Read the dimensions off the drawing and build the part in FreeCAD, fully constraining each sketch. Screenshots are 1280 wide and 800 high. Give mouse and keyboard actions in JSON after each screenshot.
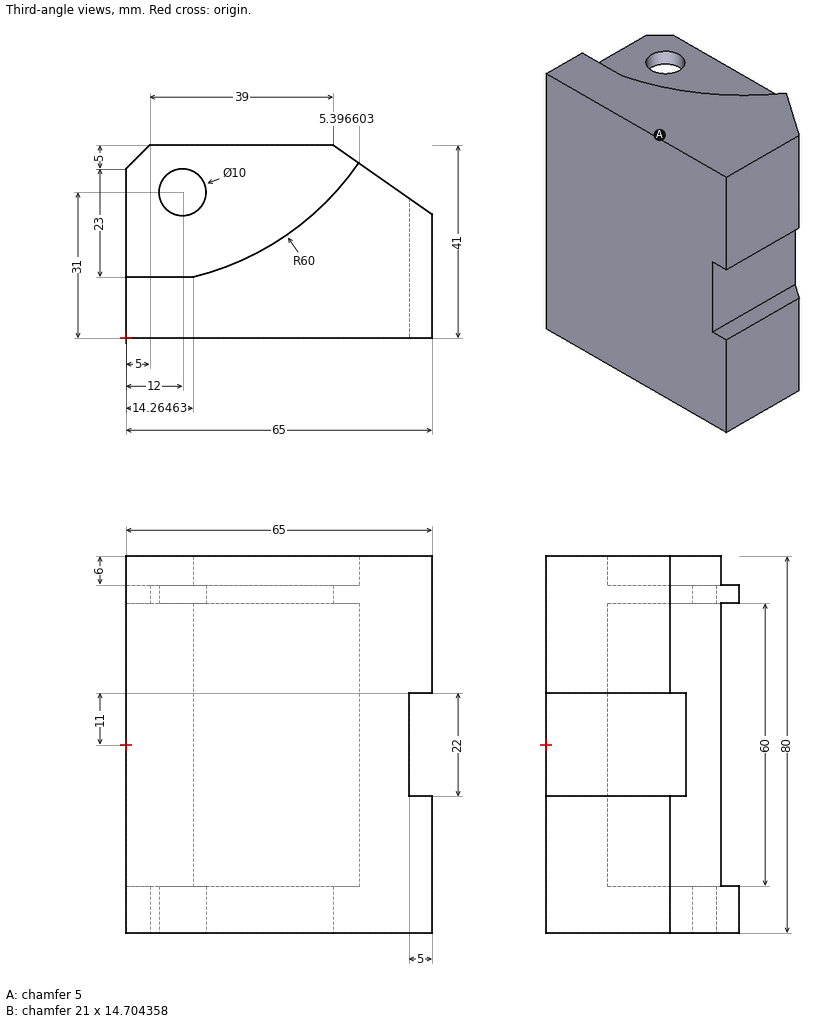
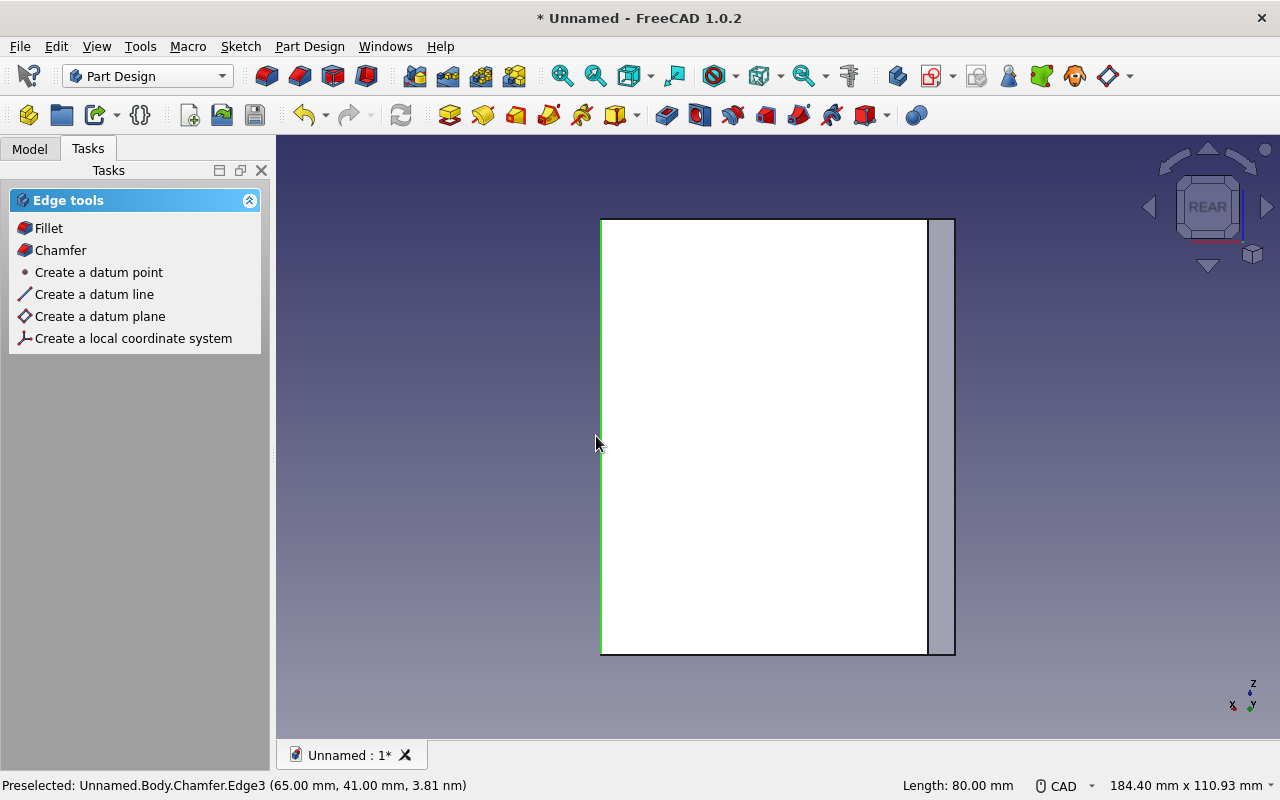
{"action": "left_click", "coordinate": [300, 76]}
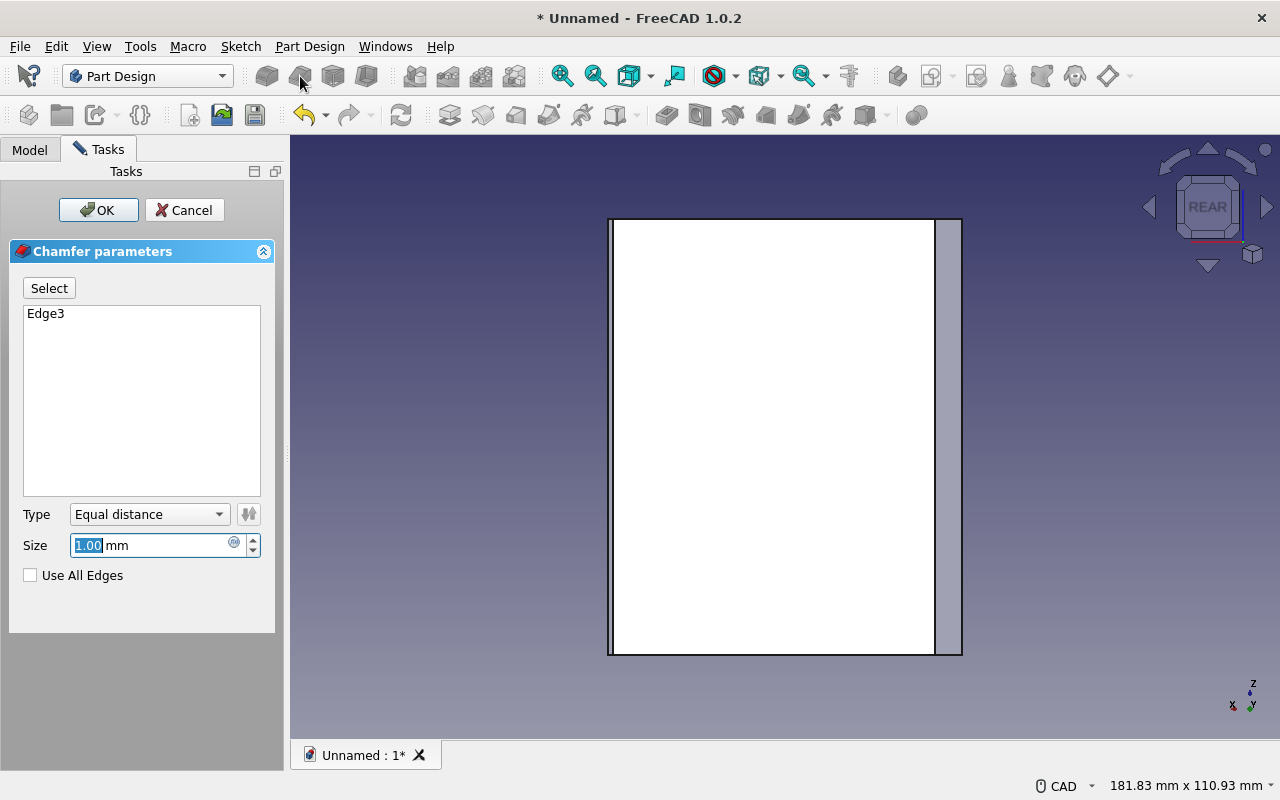
{"action": "type", "text": "21"}
{"action": "key", "text": "Tab"}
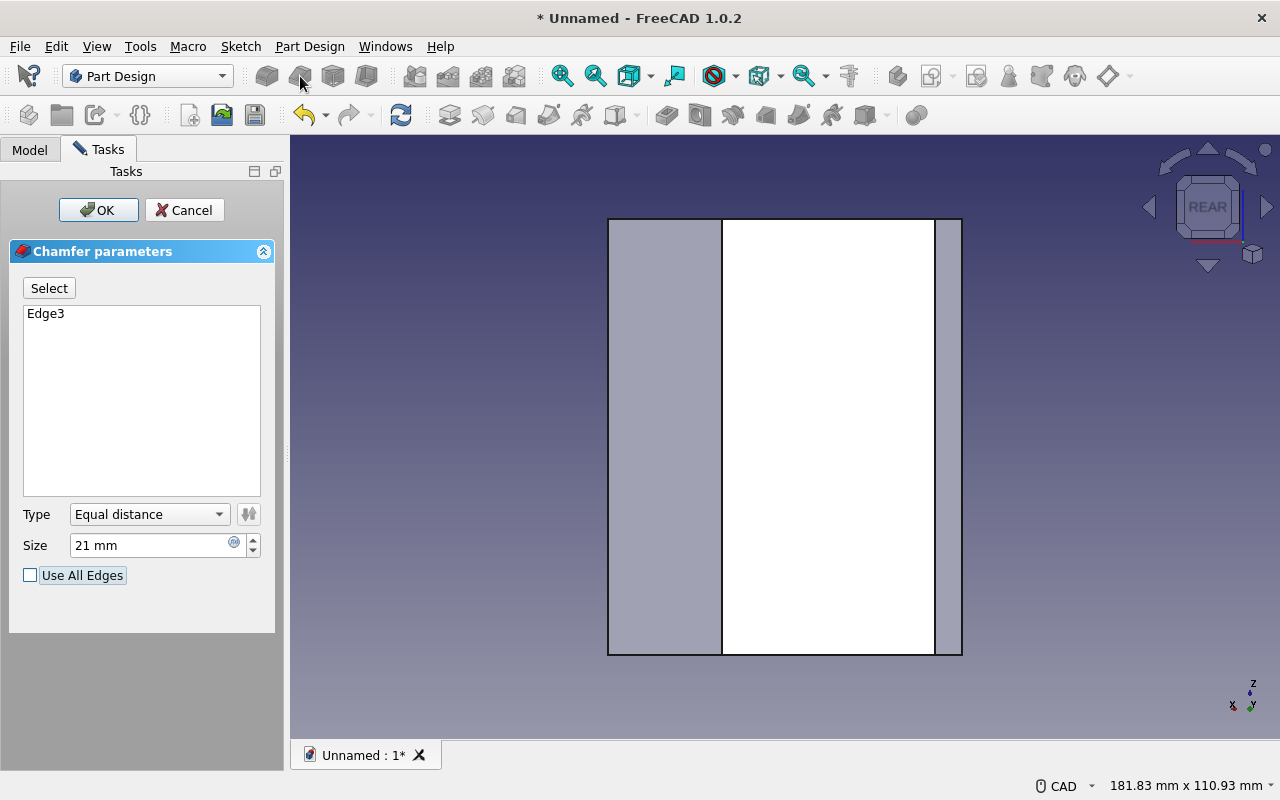
{"action": "left_click", "coordinate": [150, 514]}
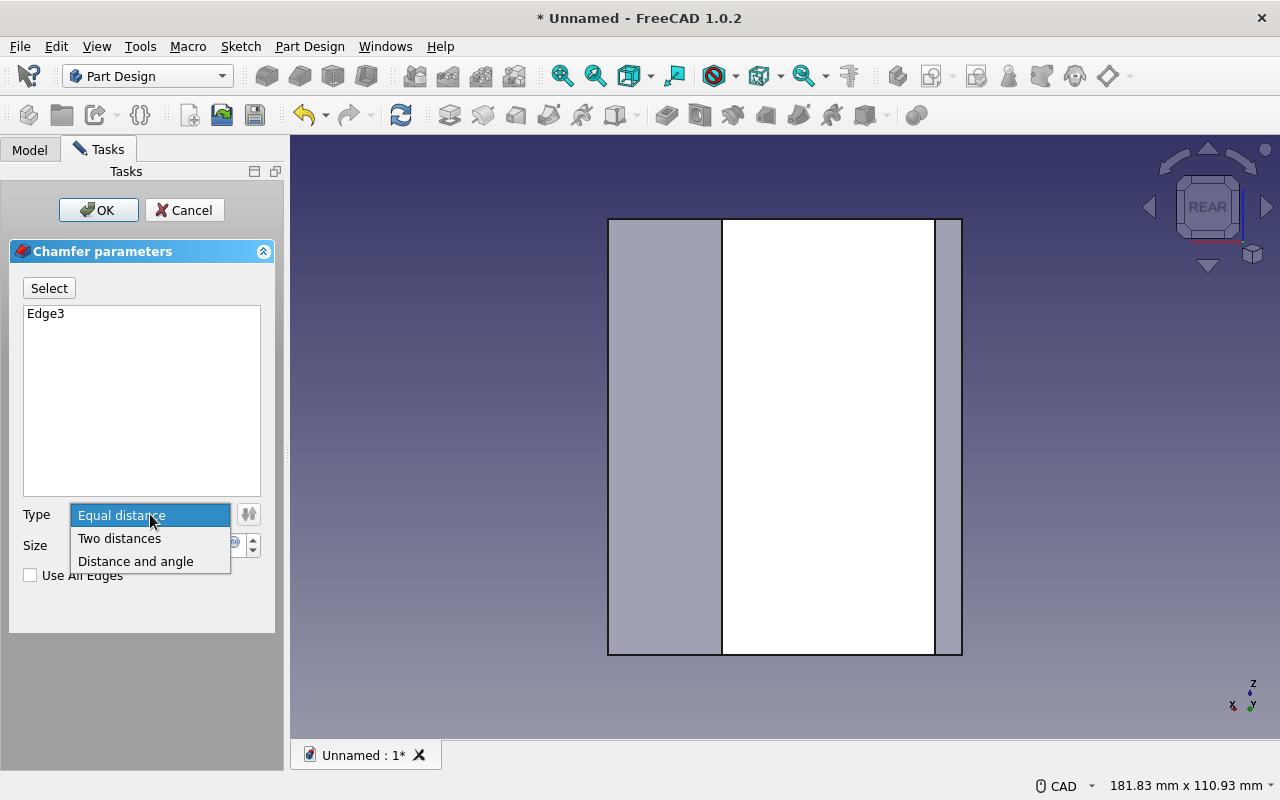
{"action": "left_click", "coordinate": [148, 538]}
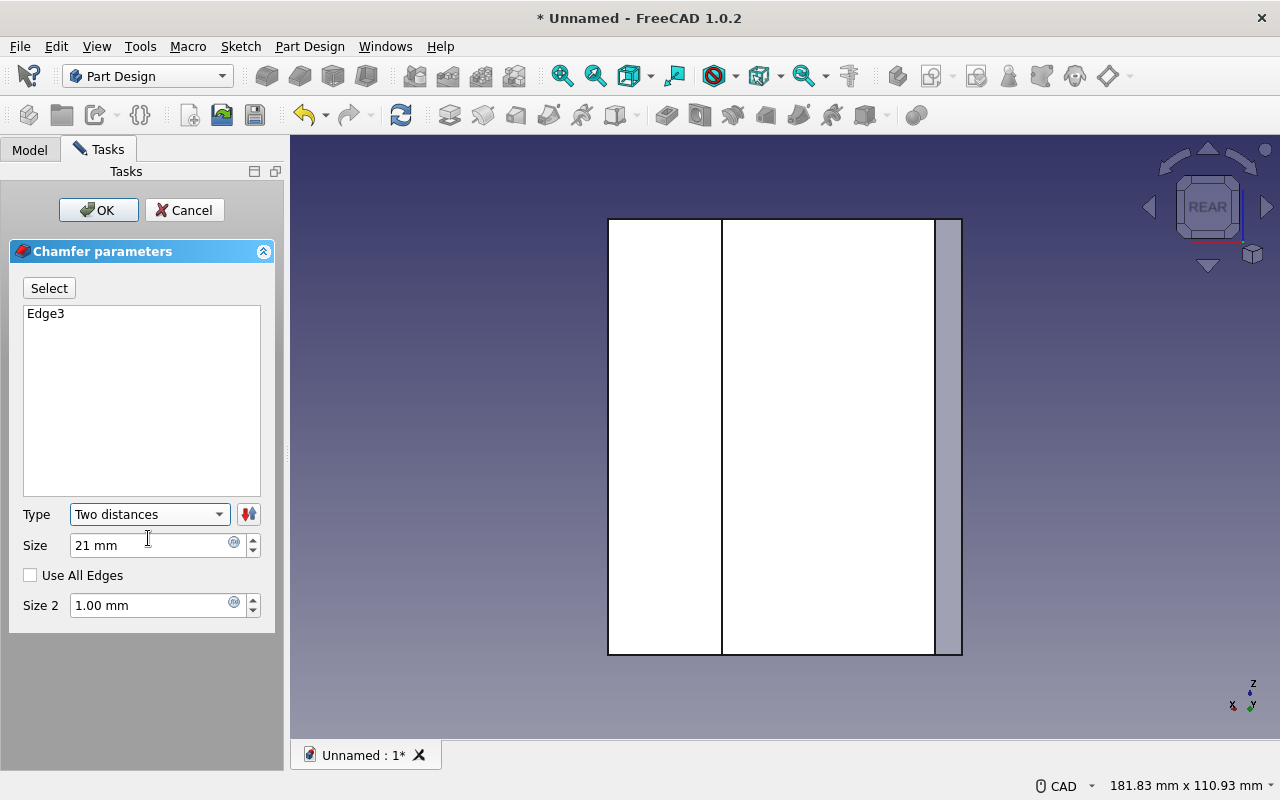
{"action": "triple_click", "coordinate": [158, 606]}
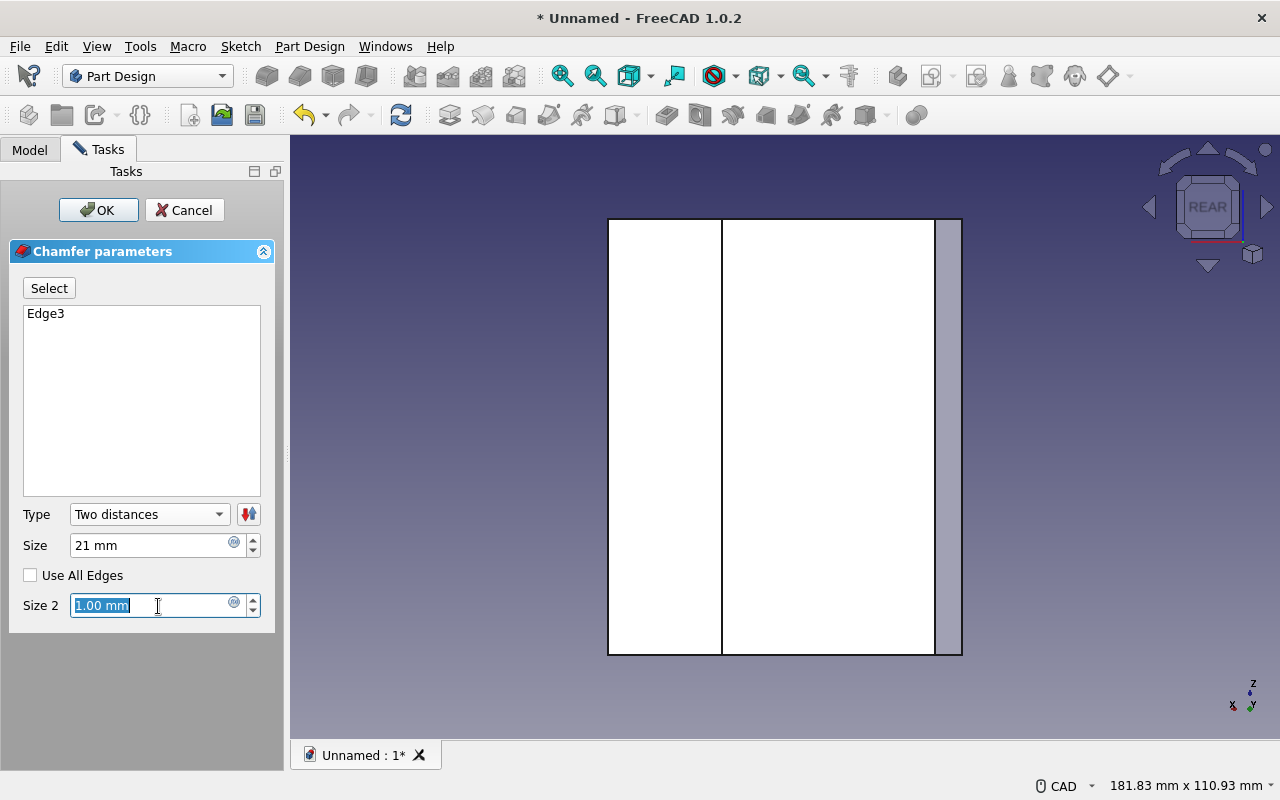
{"action": "type", "text": "14.704358"}
{"action": "key", "text": "Tab"}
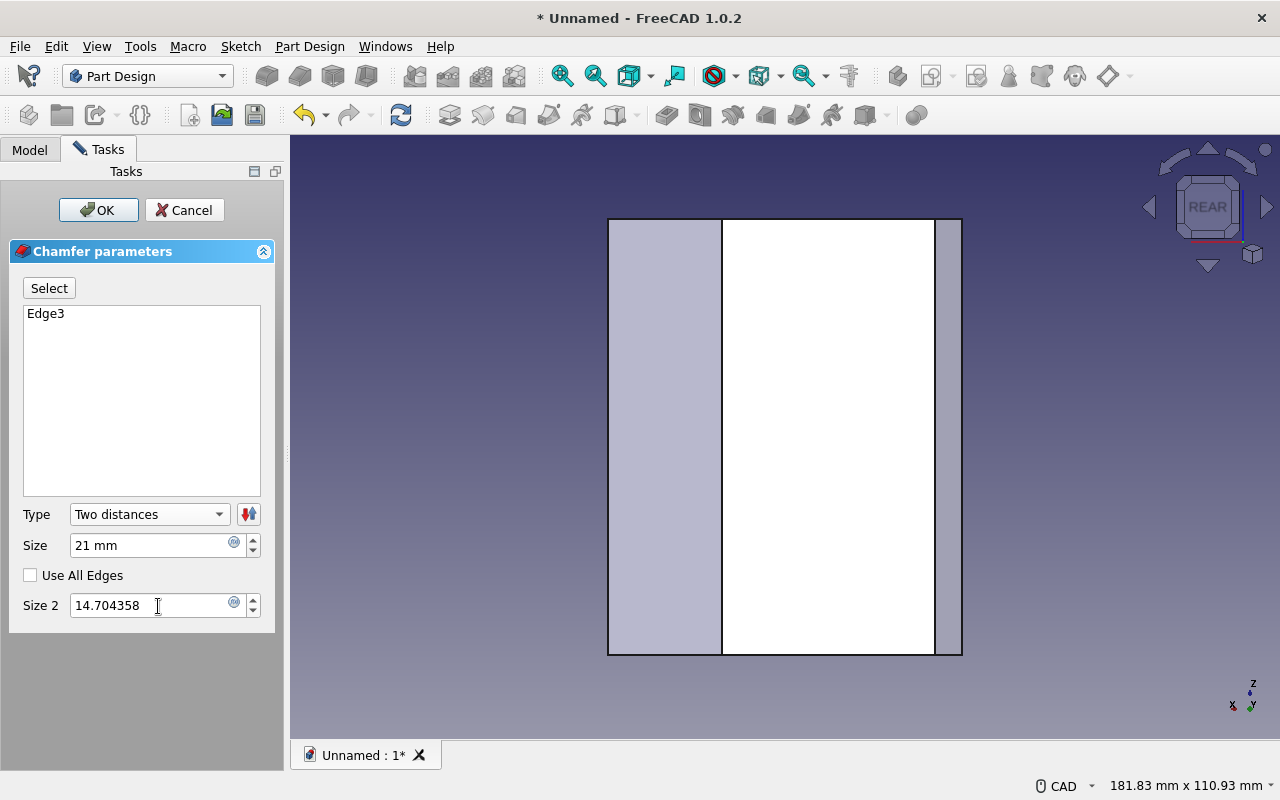
{"action": "left_click", "coordinate": [99, 210]}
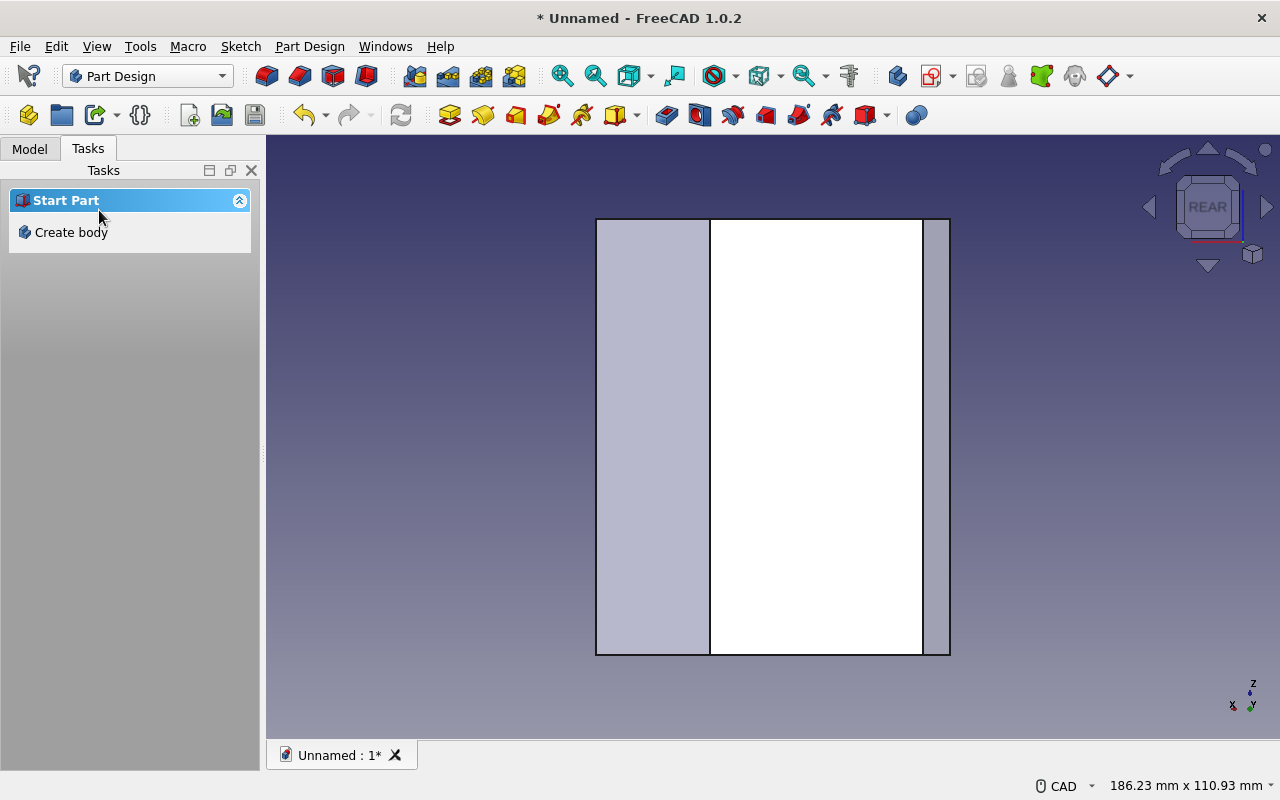
{"action": "key", "text": "0"}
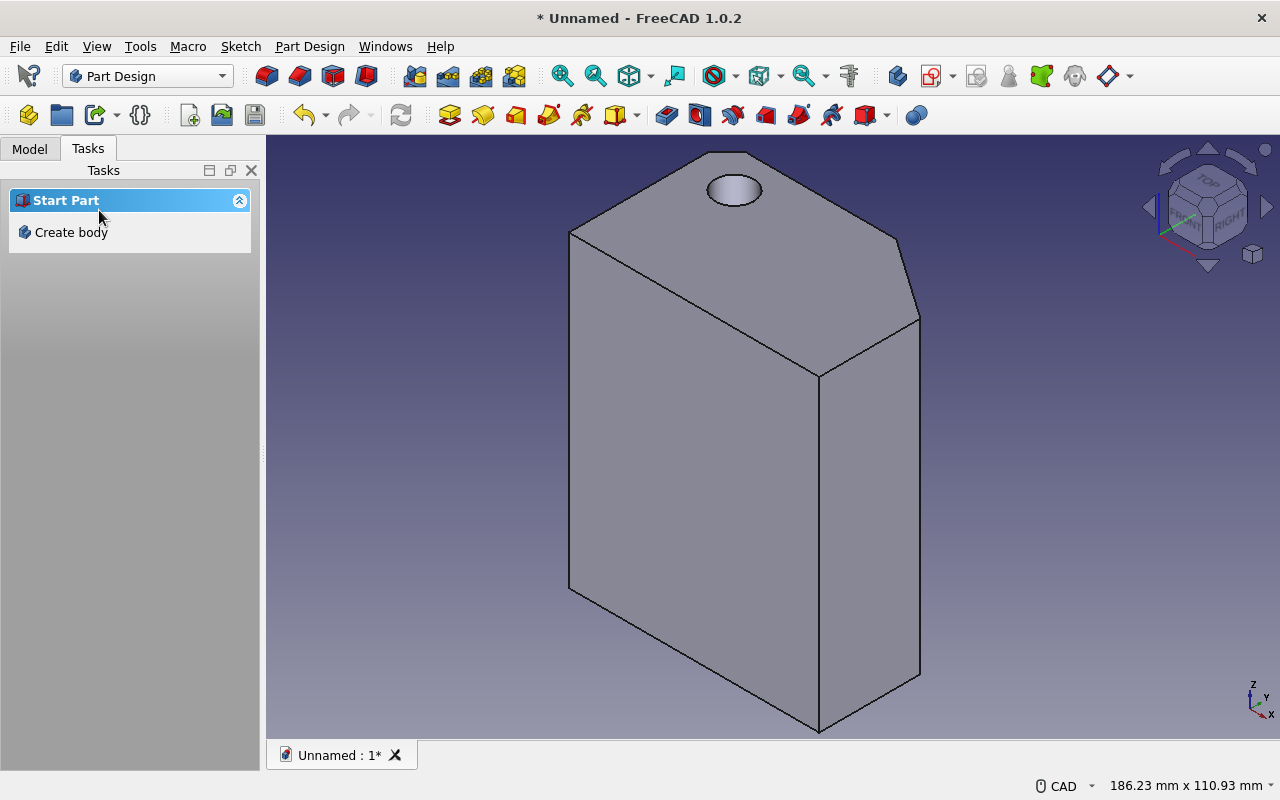
{"action": "left_click", "coordinate": [809, 279]}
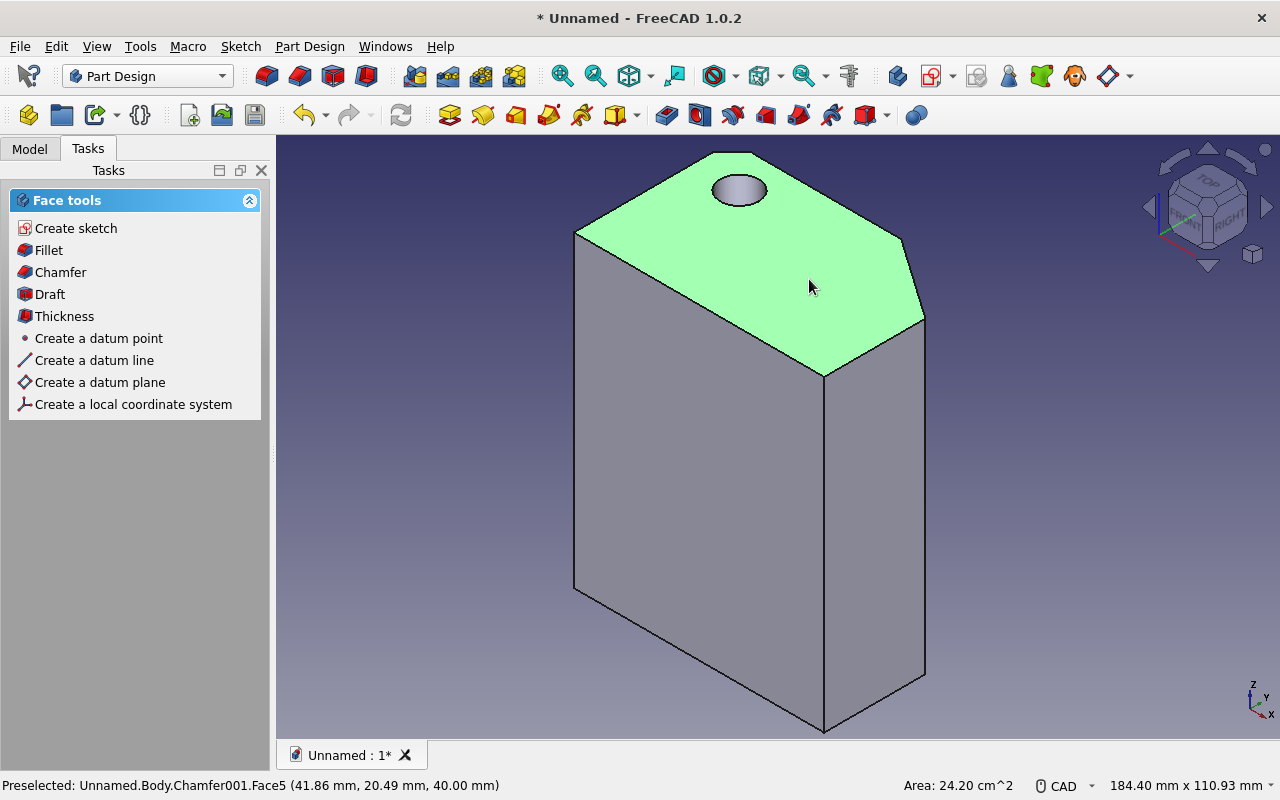
{"action": "left_click", "coordinate": [930, 76]}